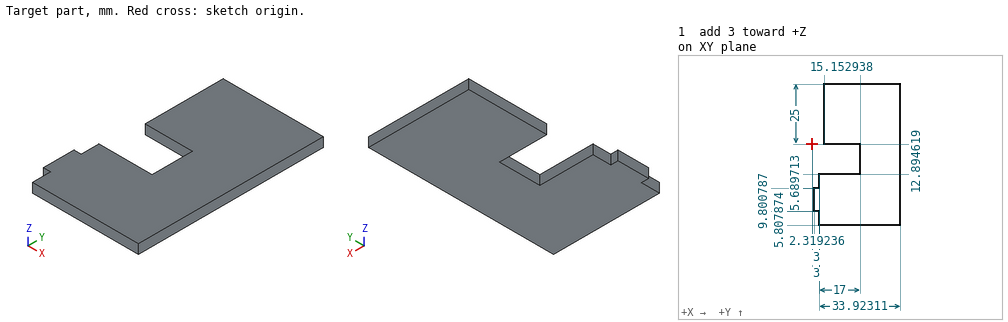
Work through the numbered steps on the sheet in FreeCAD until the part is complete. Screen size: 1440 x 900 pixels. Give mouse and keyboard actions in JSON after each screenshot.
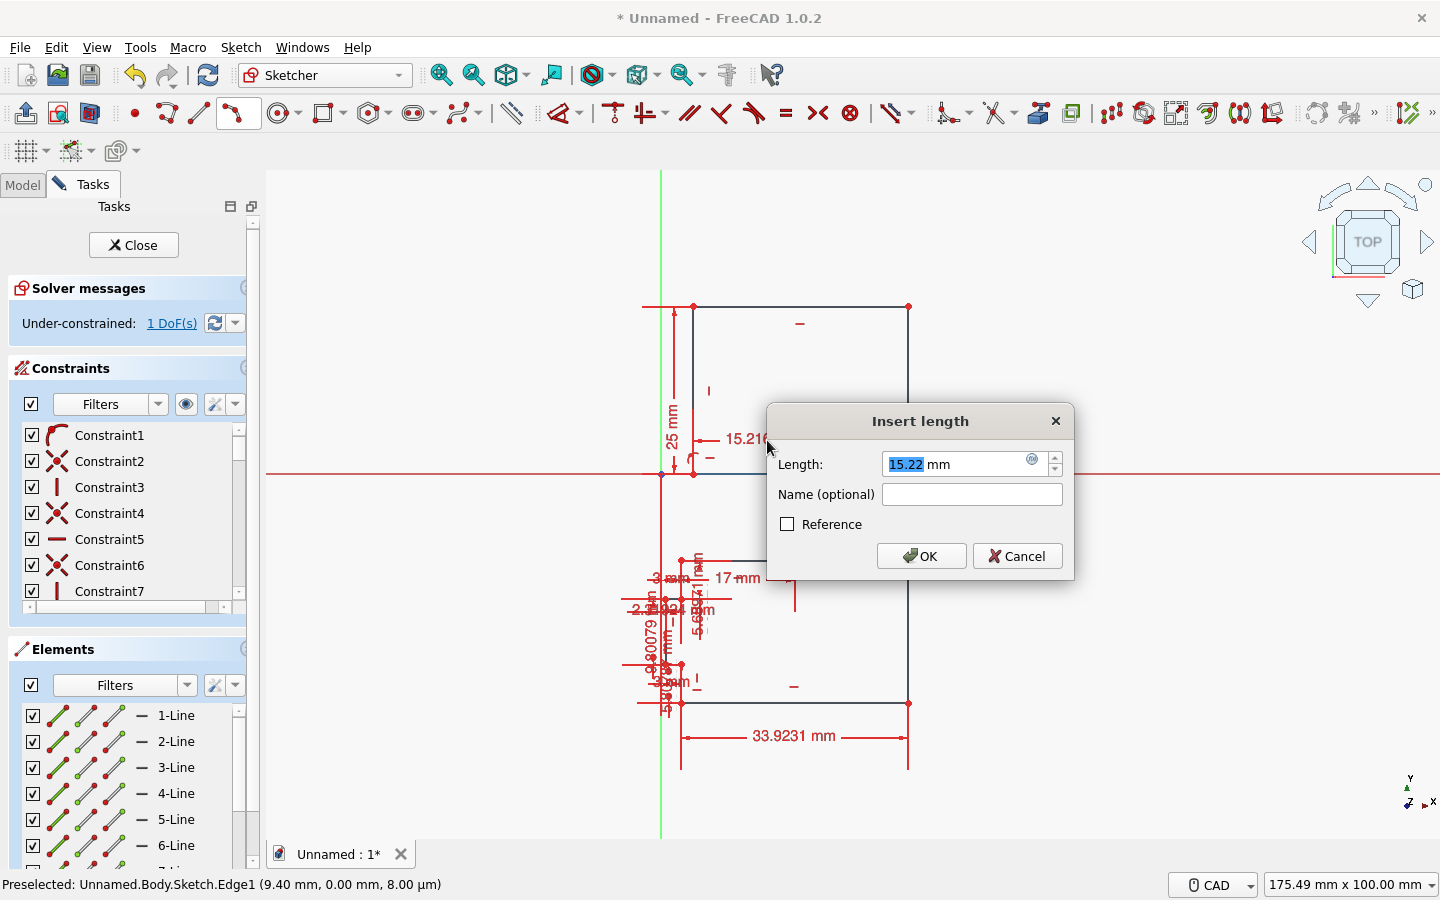
{"action": "type", "text": "15.152938"}
{"action": "key", "text": "Return"}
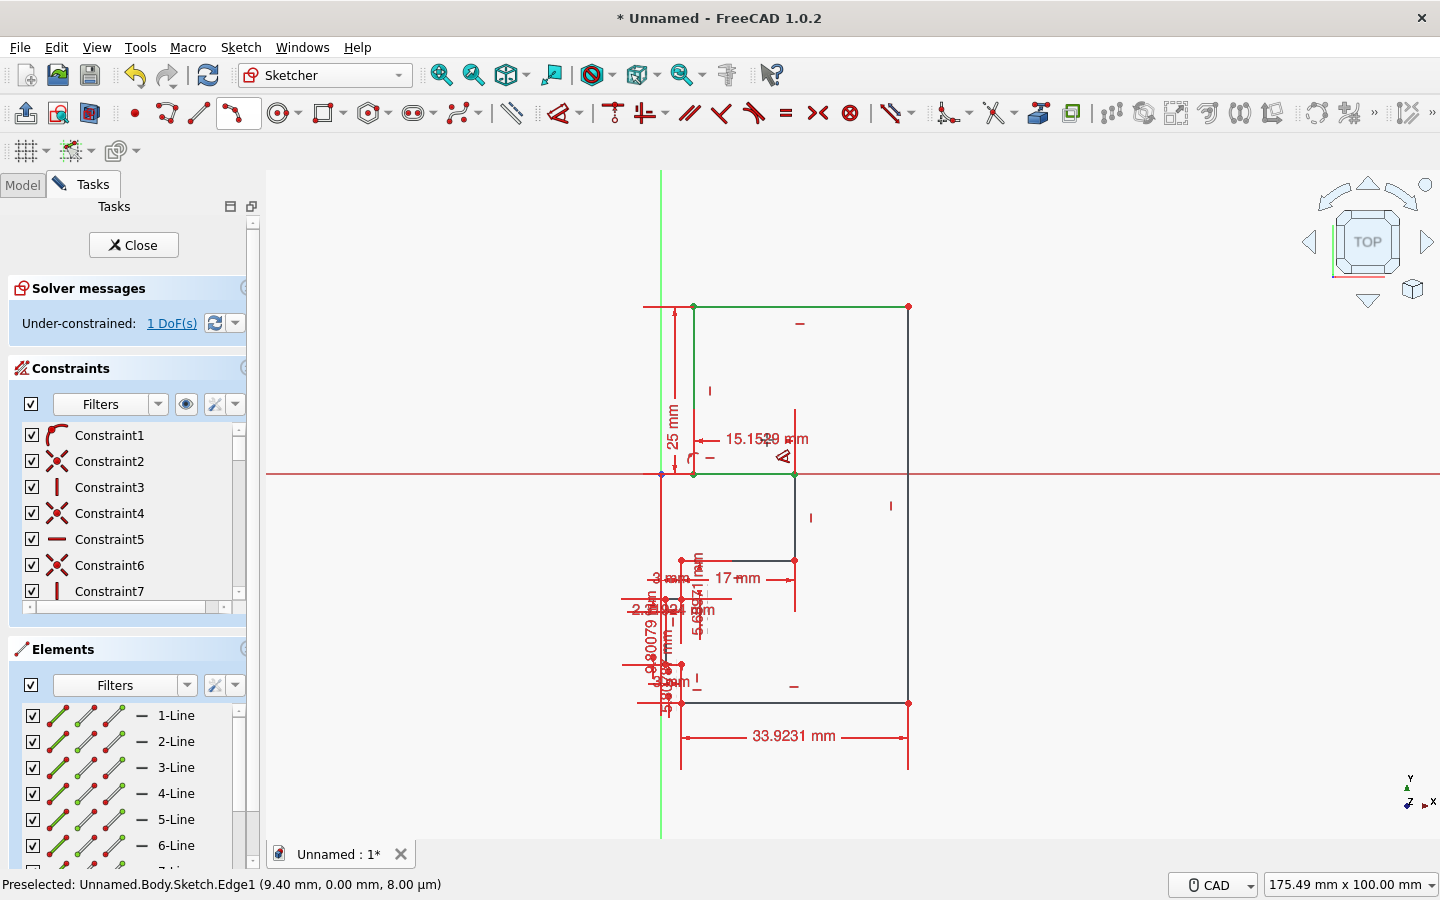
{"action": "left_click", "coordinate": [795, 500]}
{"action": "left_click", "coordinate": [829, 518]}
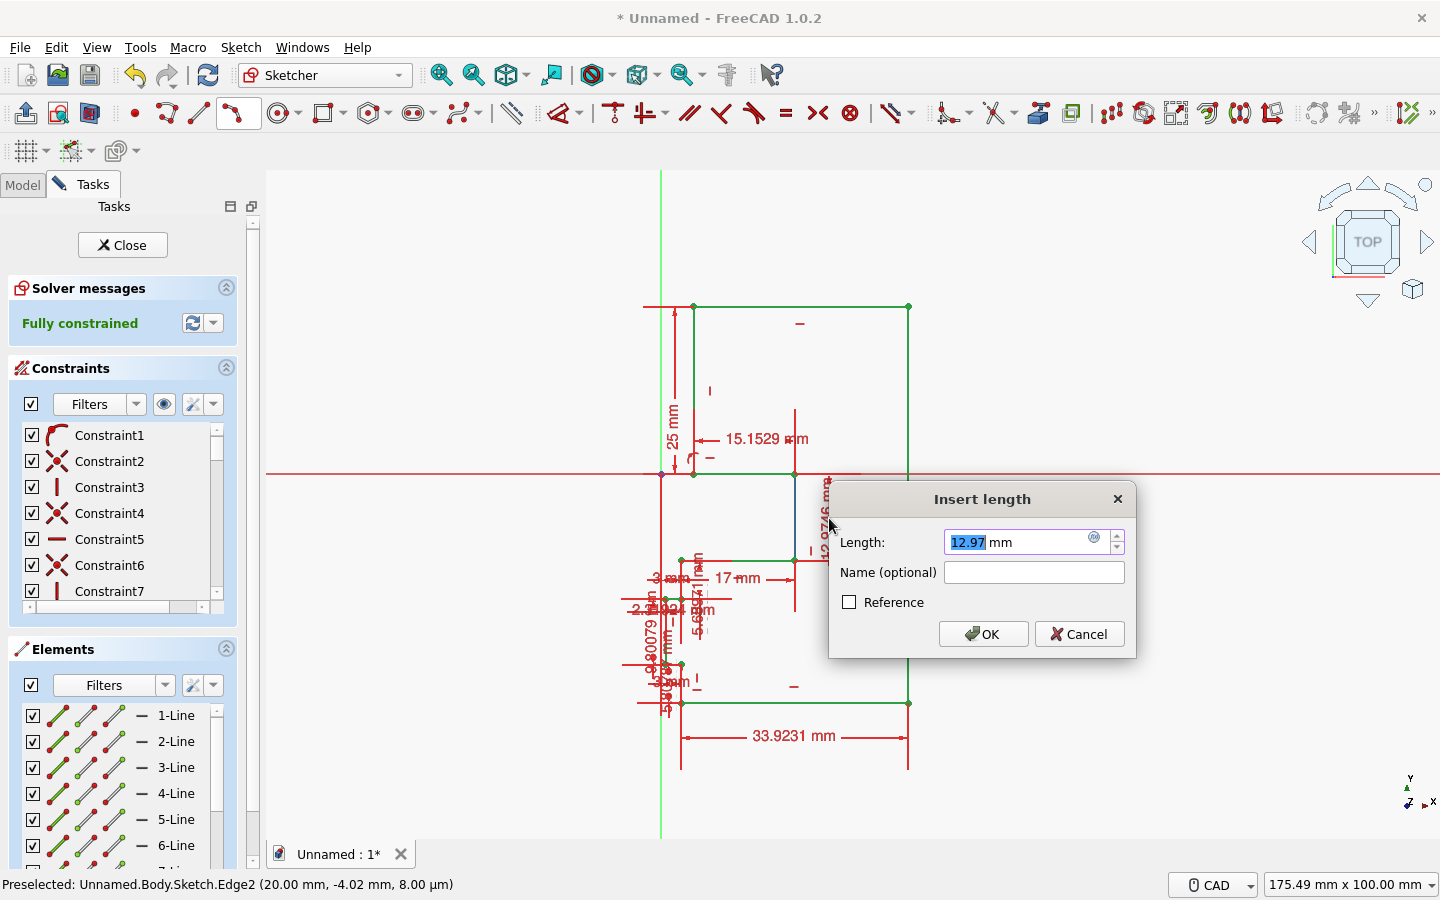
{"action": "type", "text": "12.894619"}
{"action": "key", "text": "Return"}
{"action": "key", "text": "Escape"}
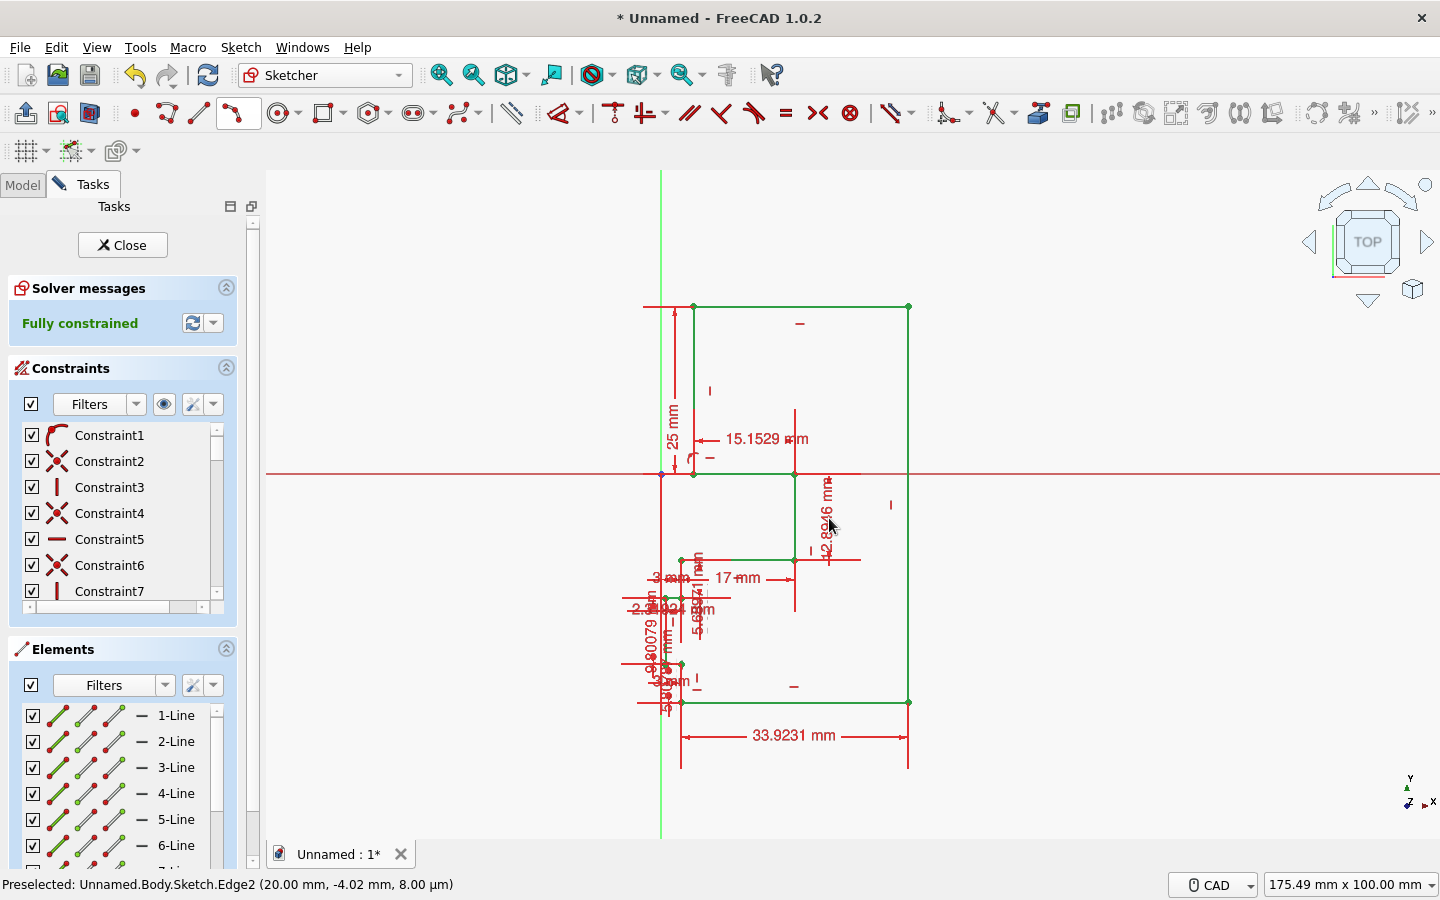
{"action": "left_click", "coordinate": [123, 245]}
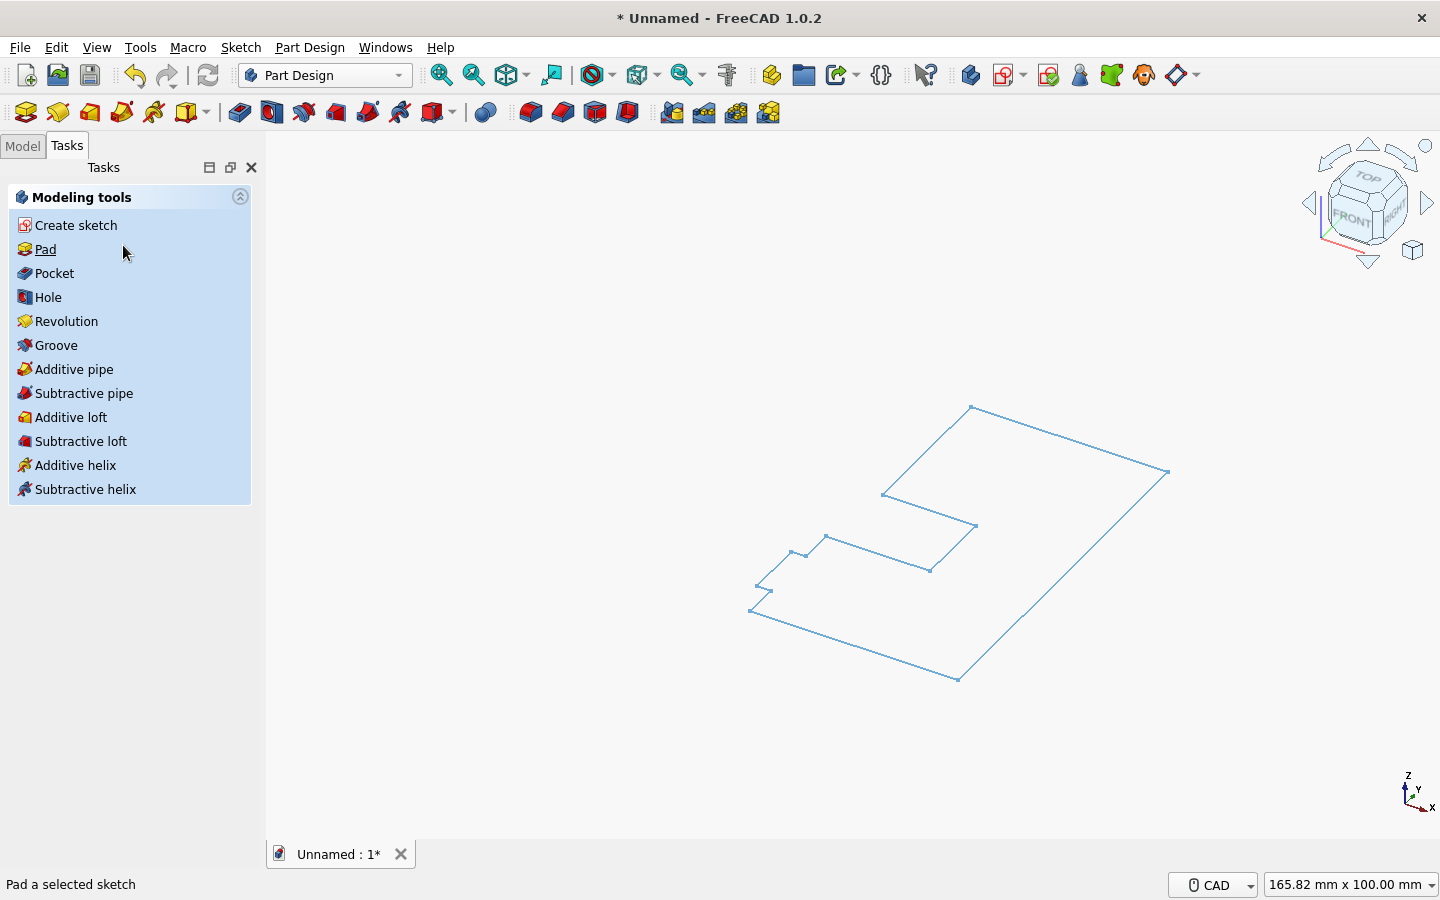
{"action": "left_click", "coordinate": [26, 112]}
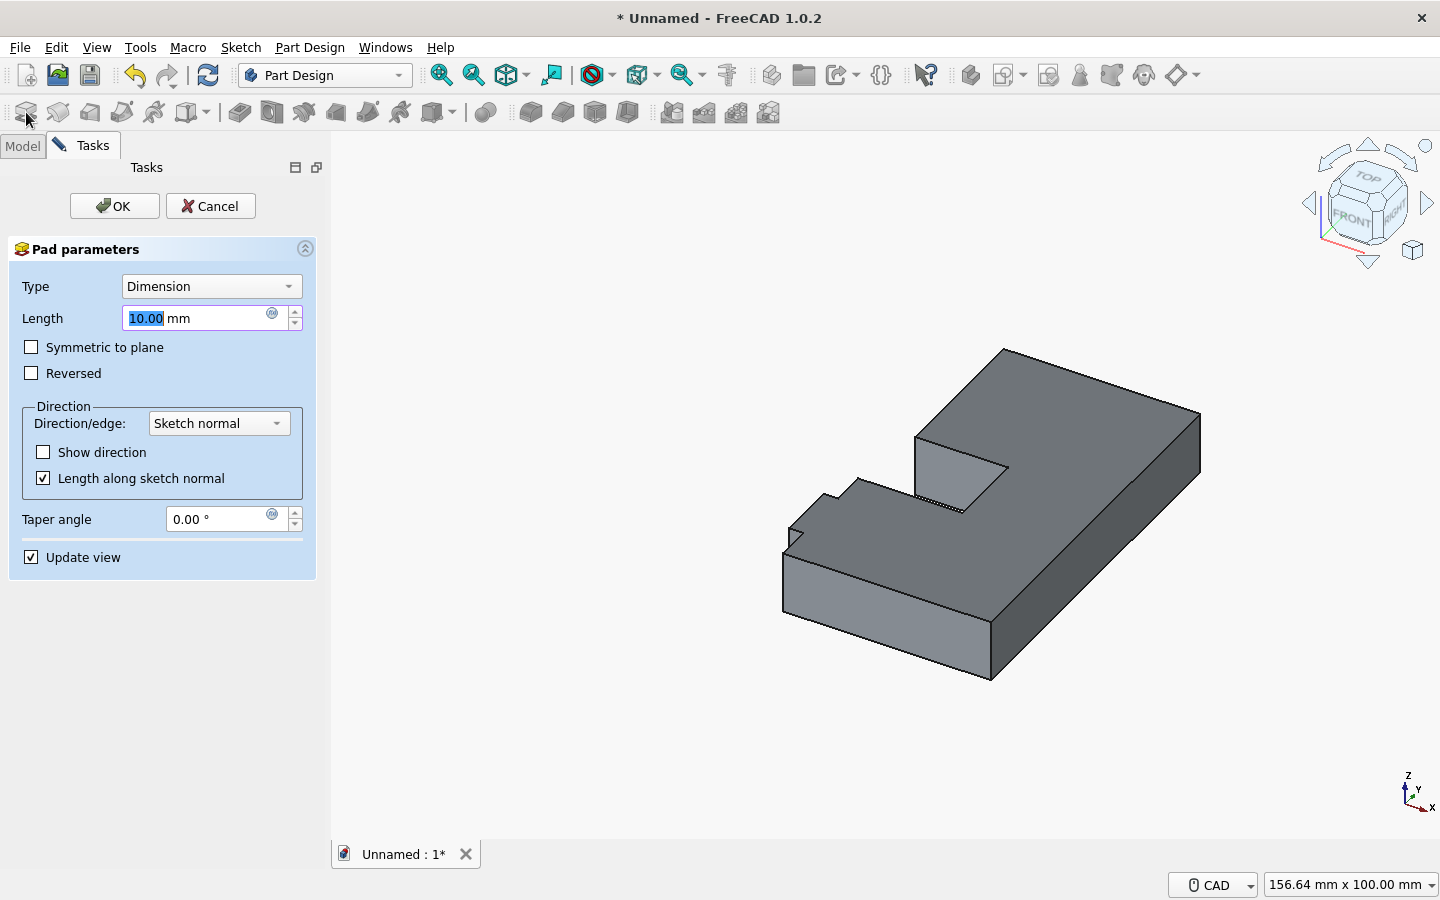
{"action": "type", "text": "3"}
{"action": "key", "text": "Tab"}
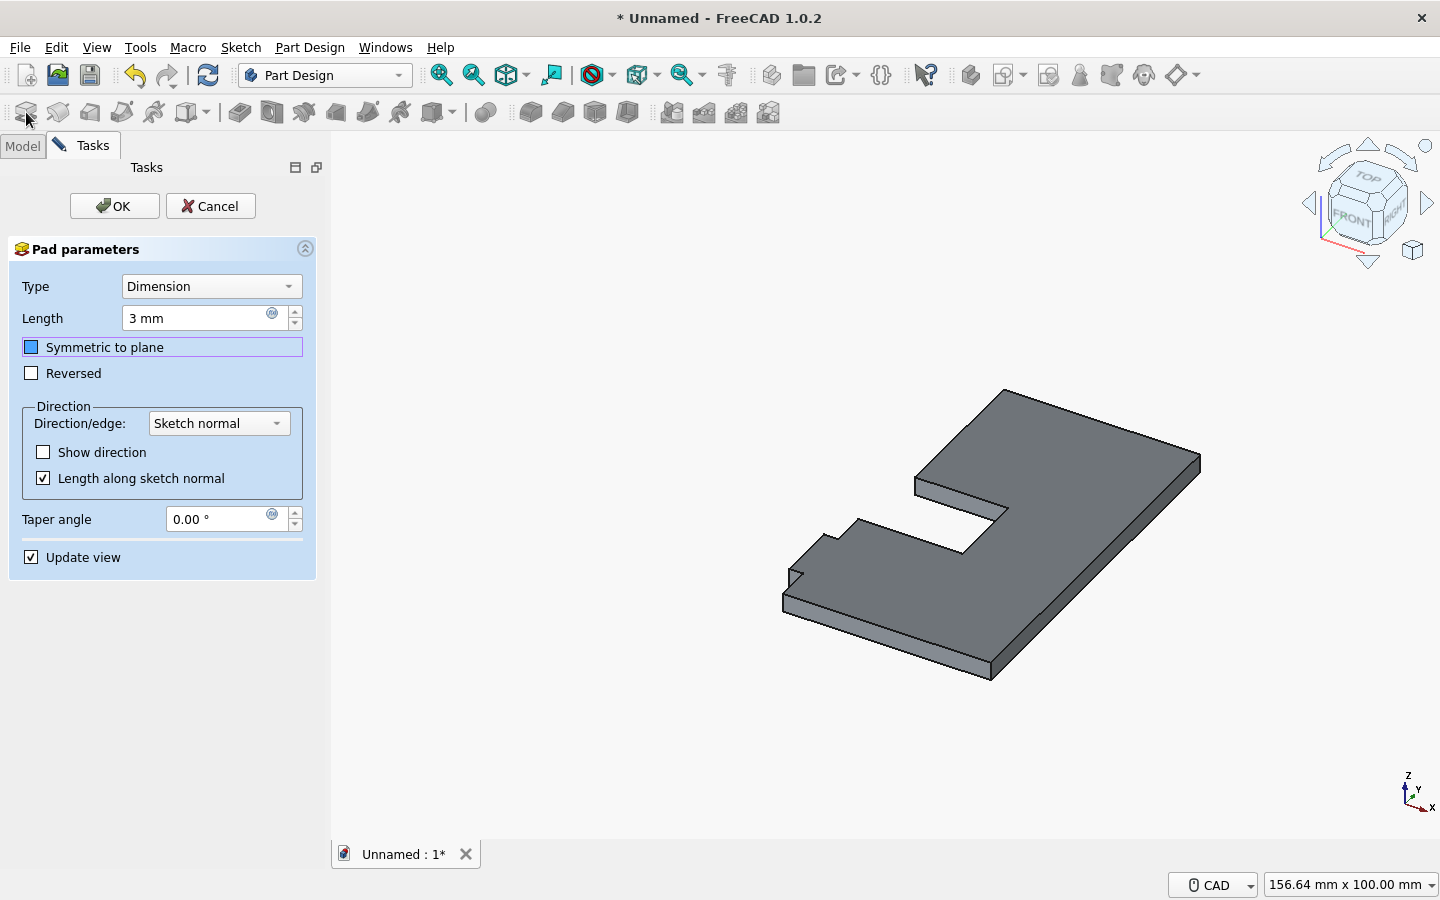
{"action": "left_click", "coordinate": [115, 206]}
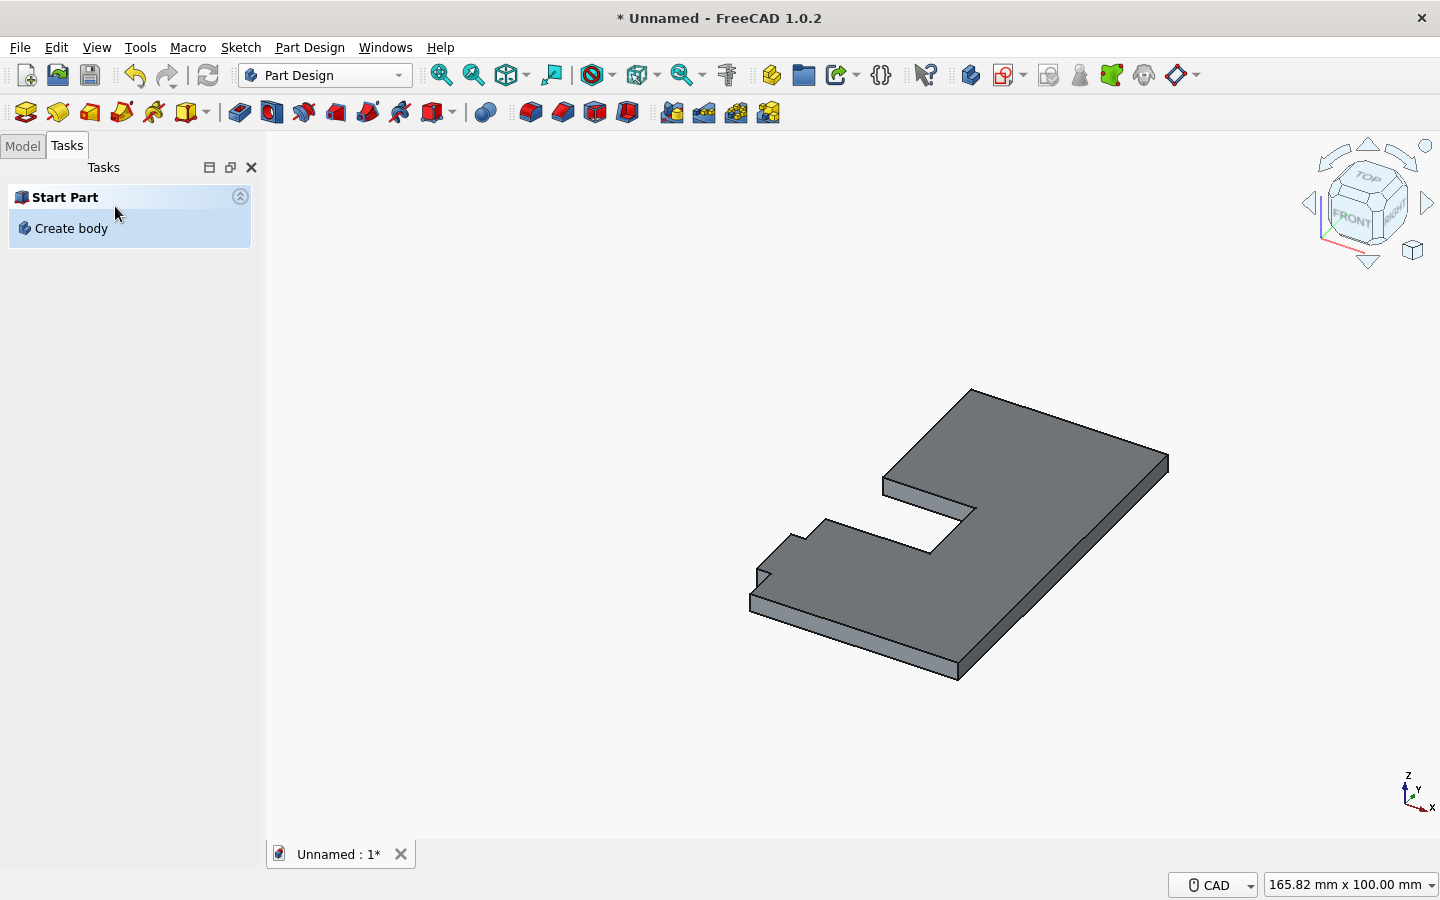
{"action": "key", "text": "0"}